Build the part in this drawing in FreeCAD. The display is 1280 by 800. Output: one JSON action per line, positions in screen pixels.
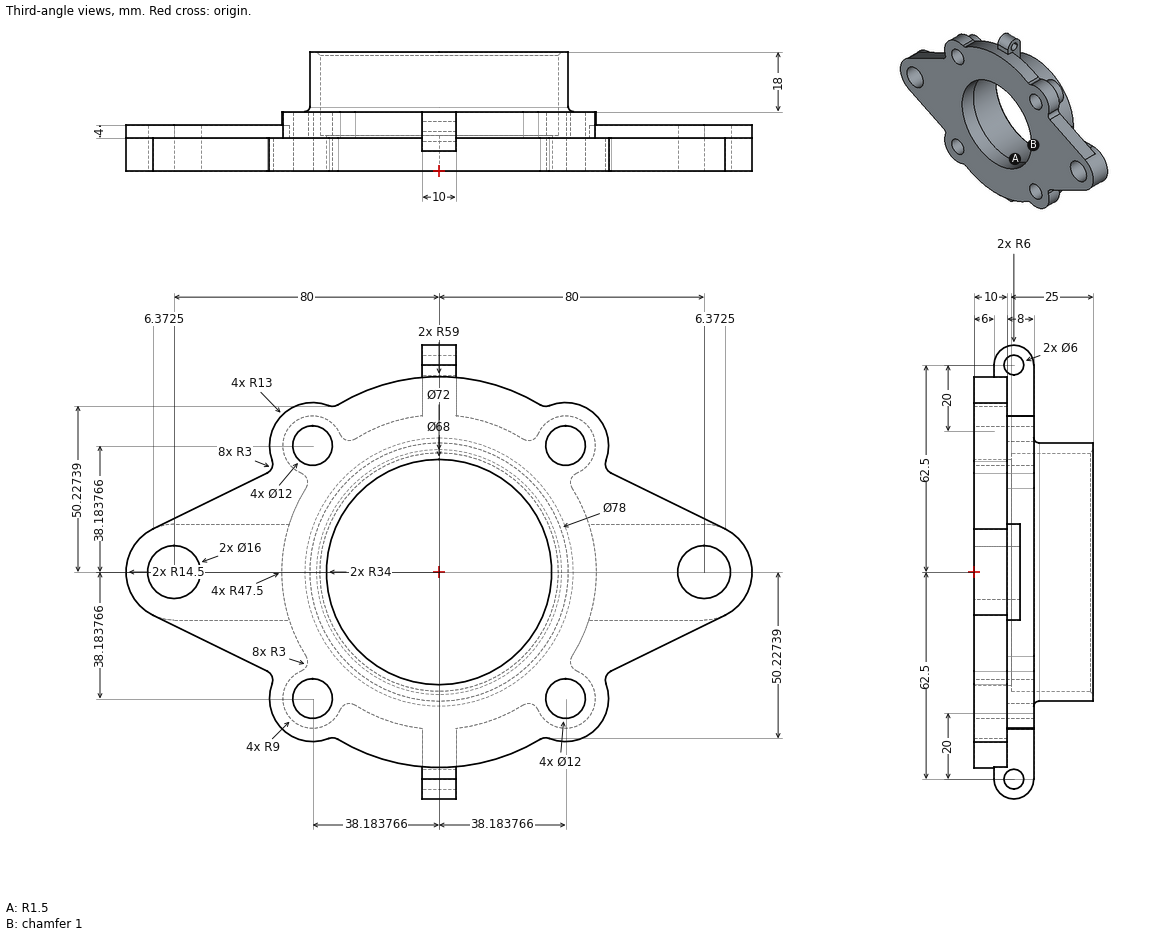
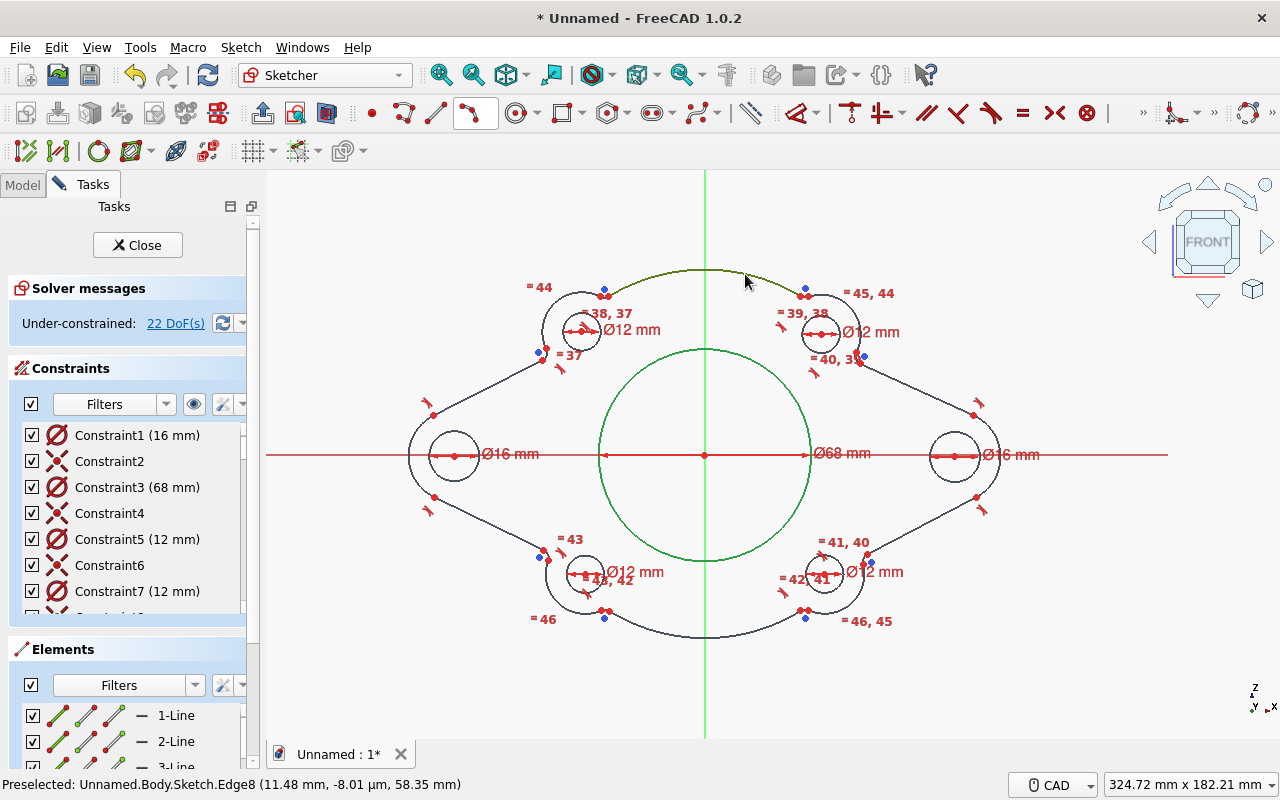
{"action": "left_click", "coordinate": [665, 634]}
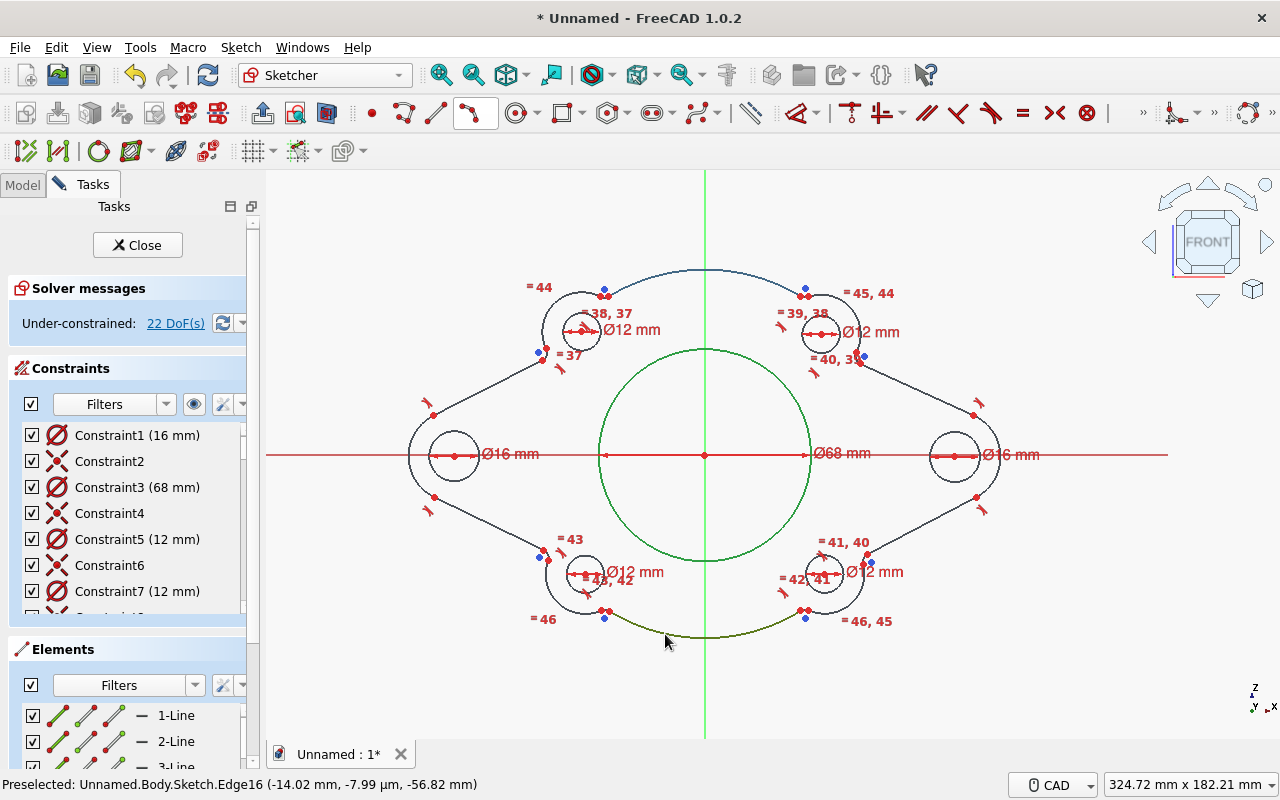
{"action": "left_click", "coordinate": [1024, 114]}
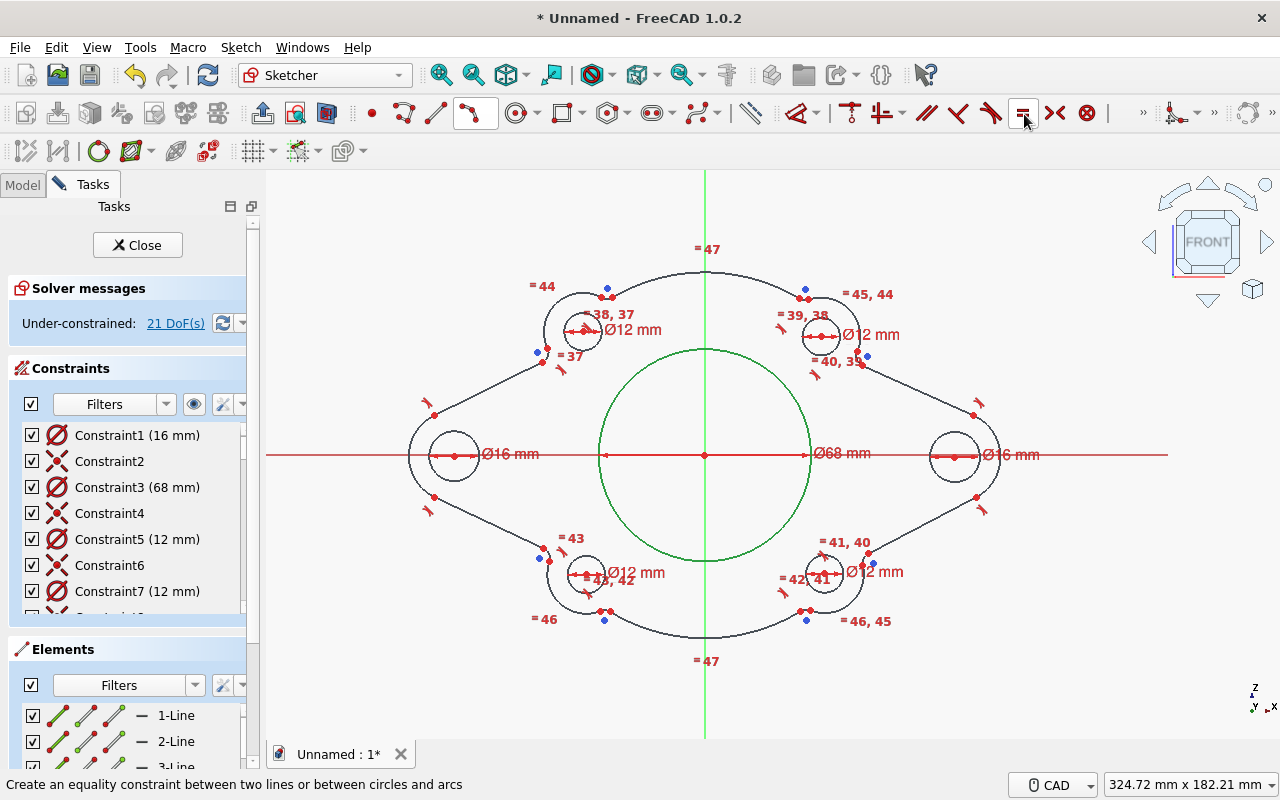
{"action": "left_click", "coordinate": [997, 475]}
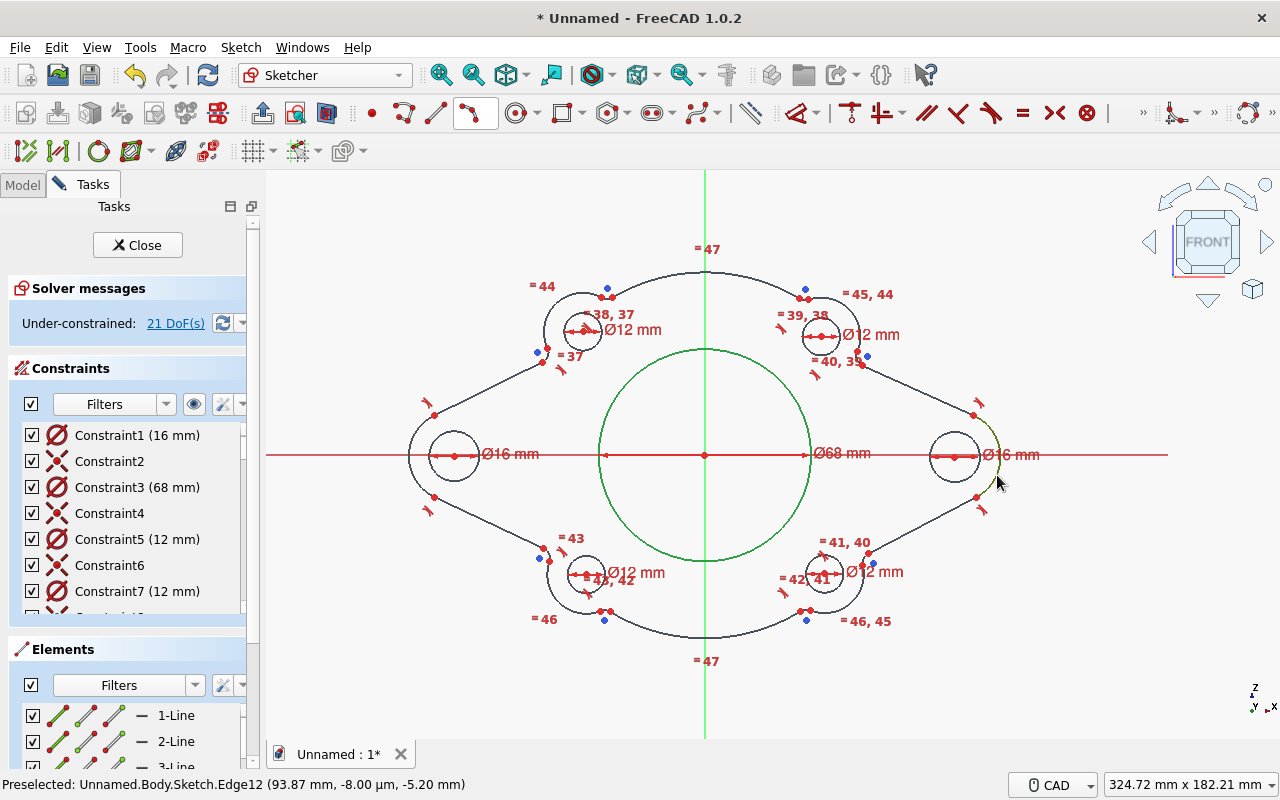
{"action": "left_click", "coordinate": [413, 437]}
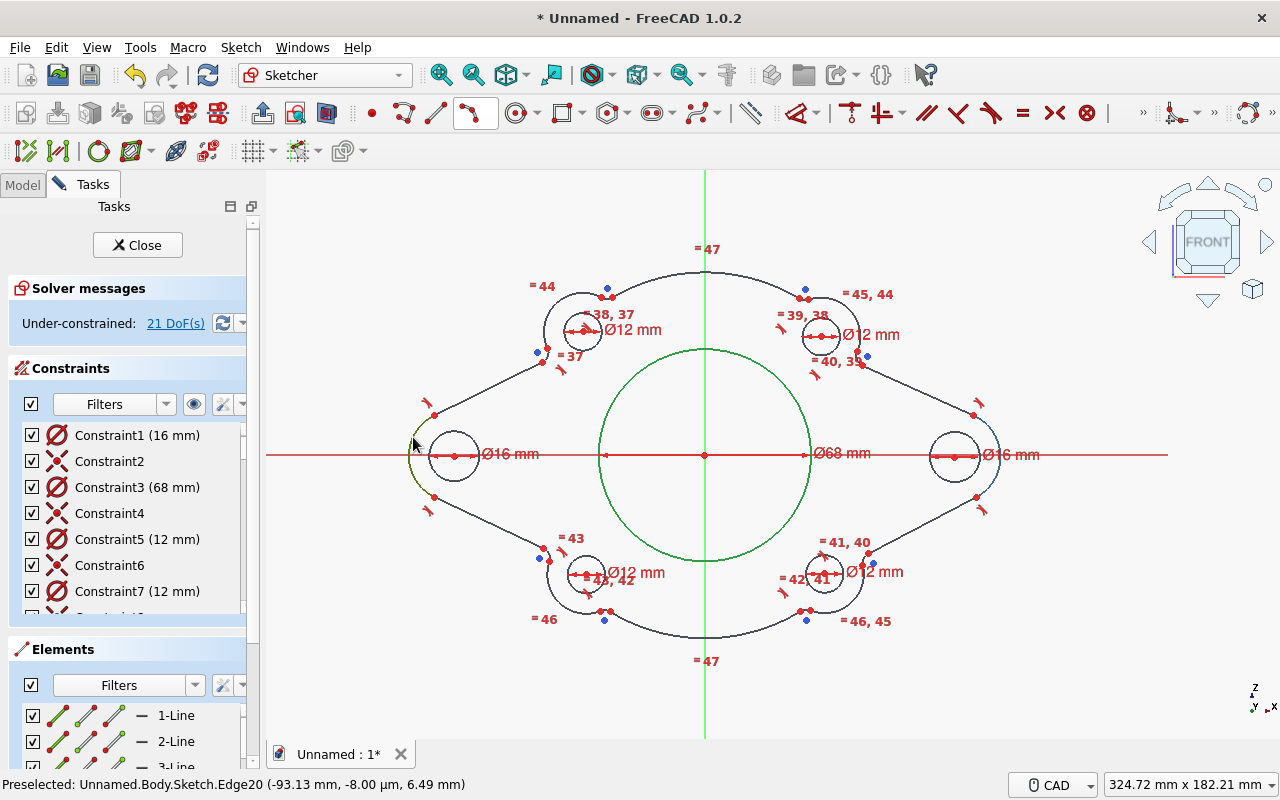
{"action": "left_click", "coordinate": [1024, 114]}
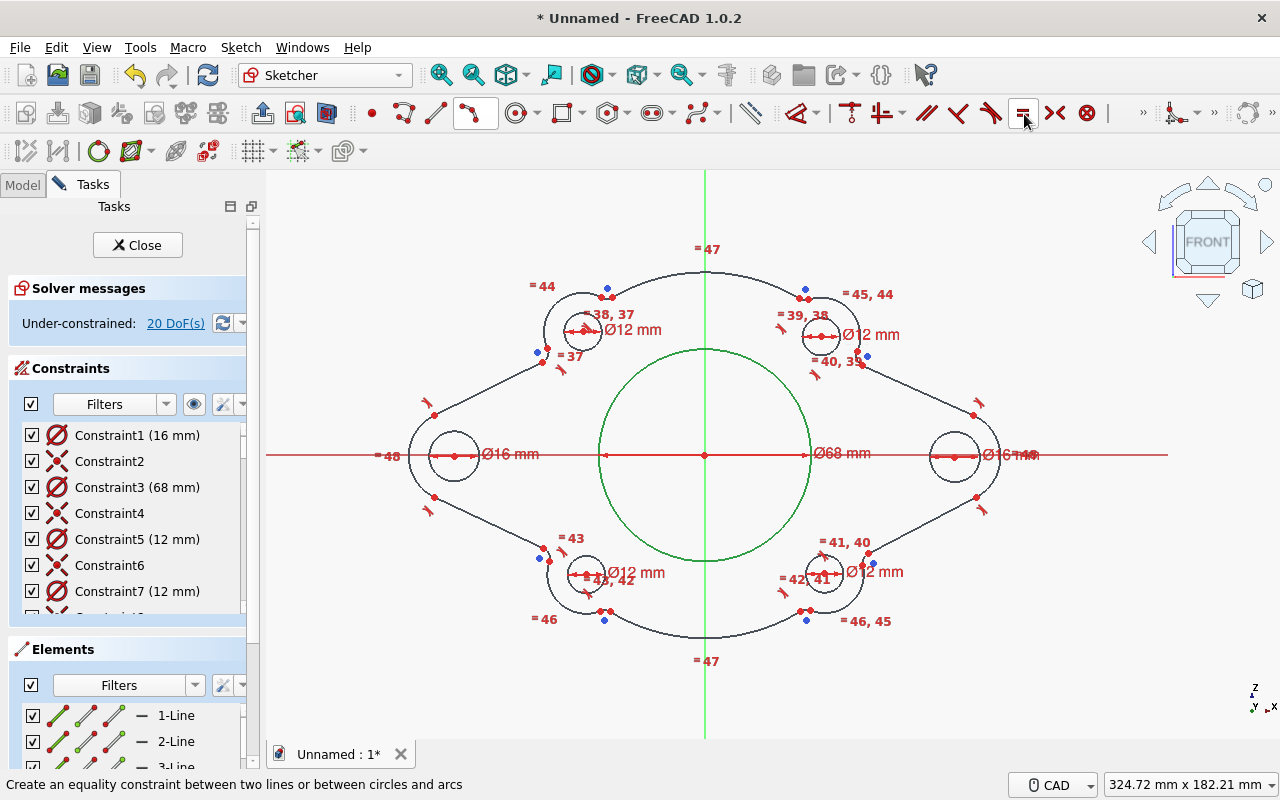
{"action": "left_click", "coordinate": [955, 457]}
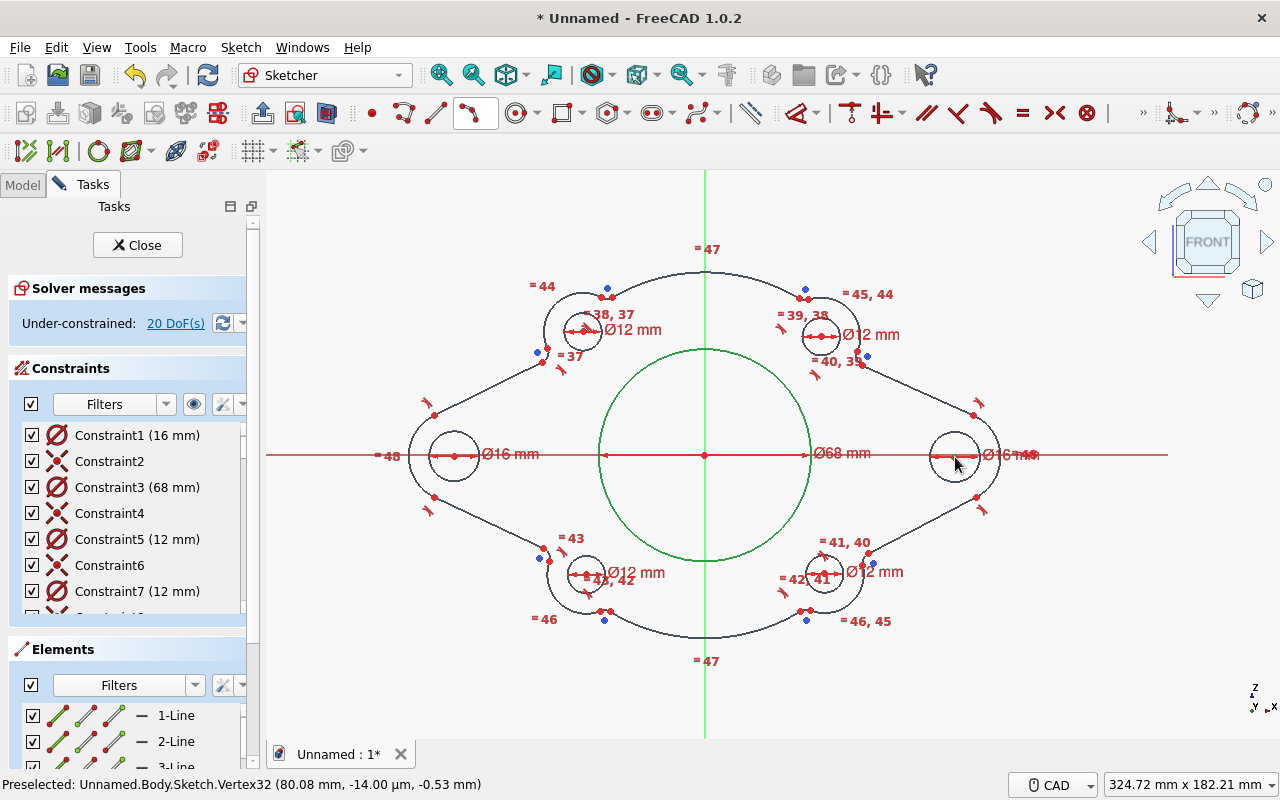
{"action": "left_click", "coordinate": [353, 455]}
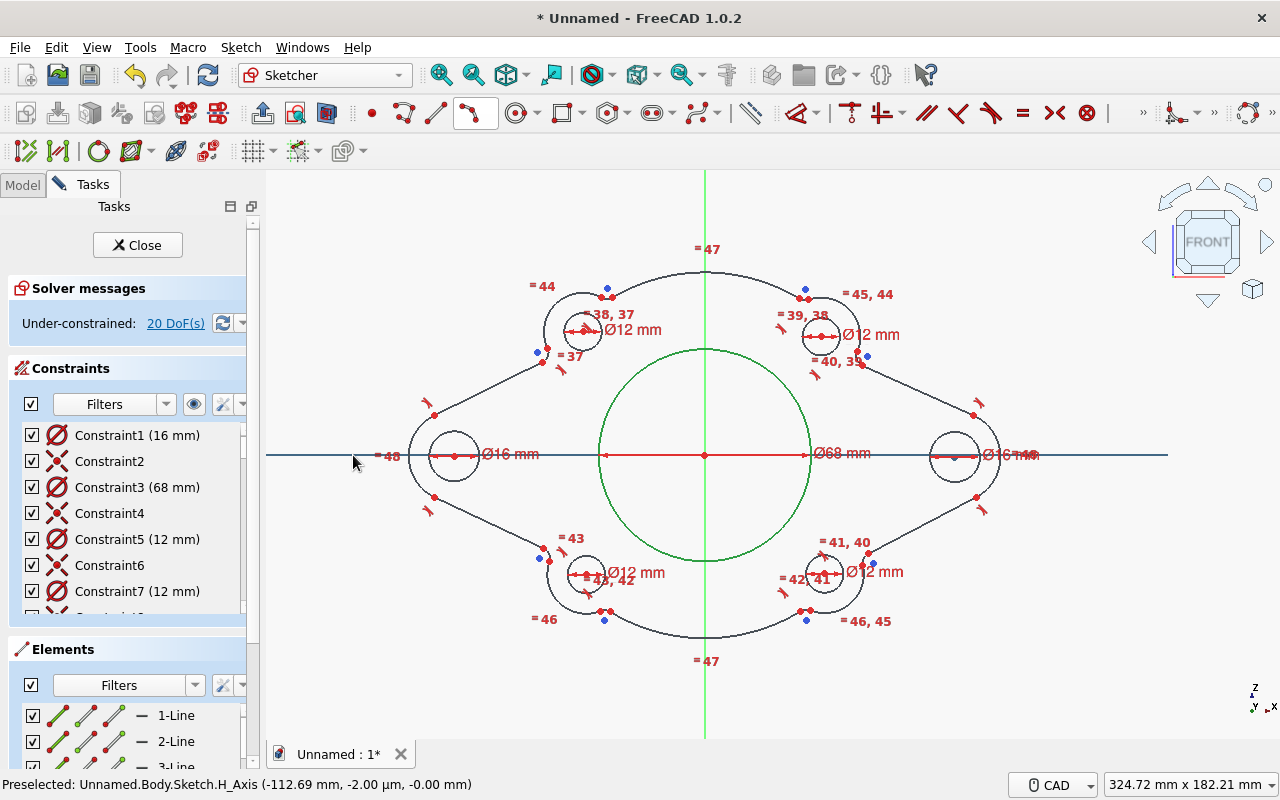
{"action": "left_click", "coordinate": [850, 114]}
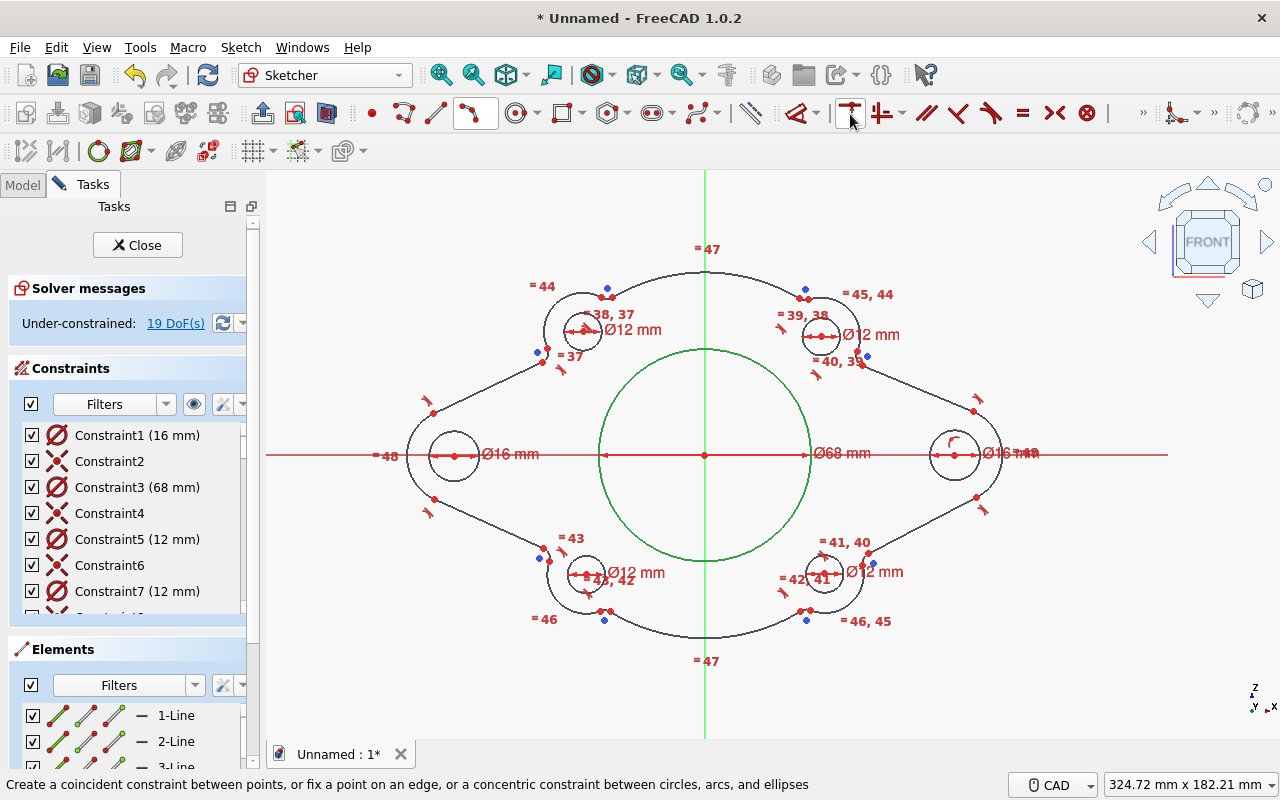
{"action": "left_click", "coordinate": [454, 456]}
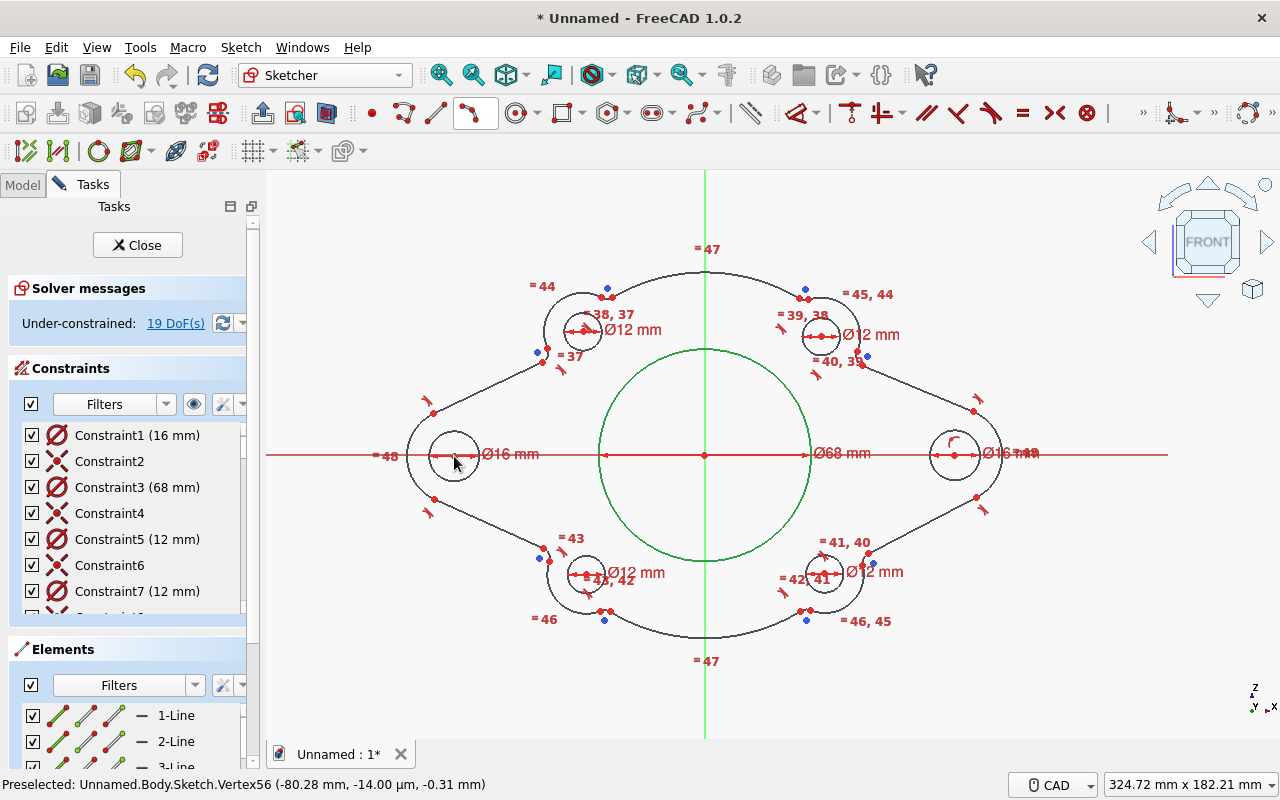
{"action": "left_click", "coordinate": [353, 455]}